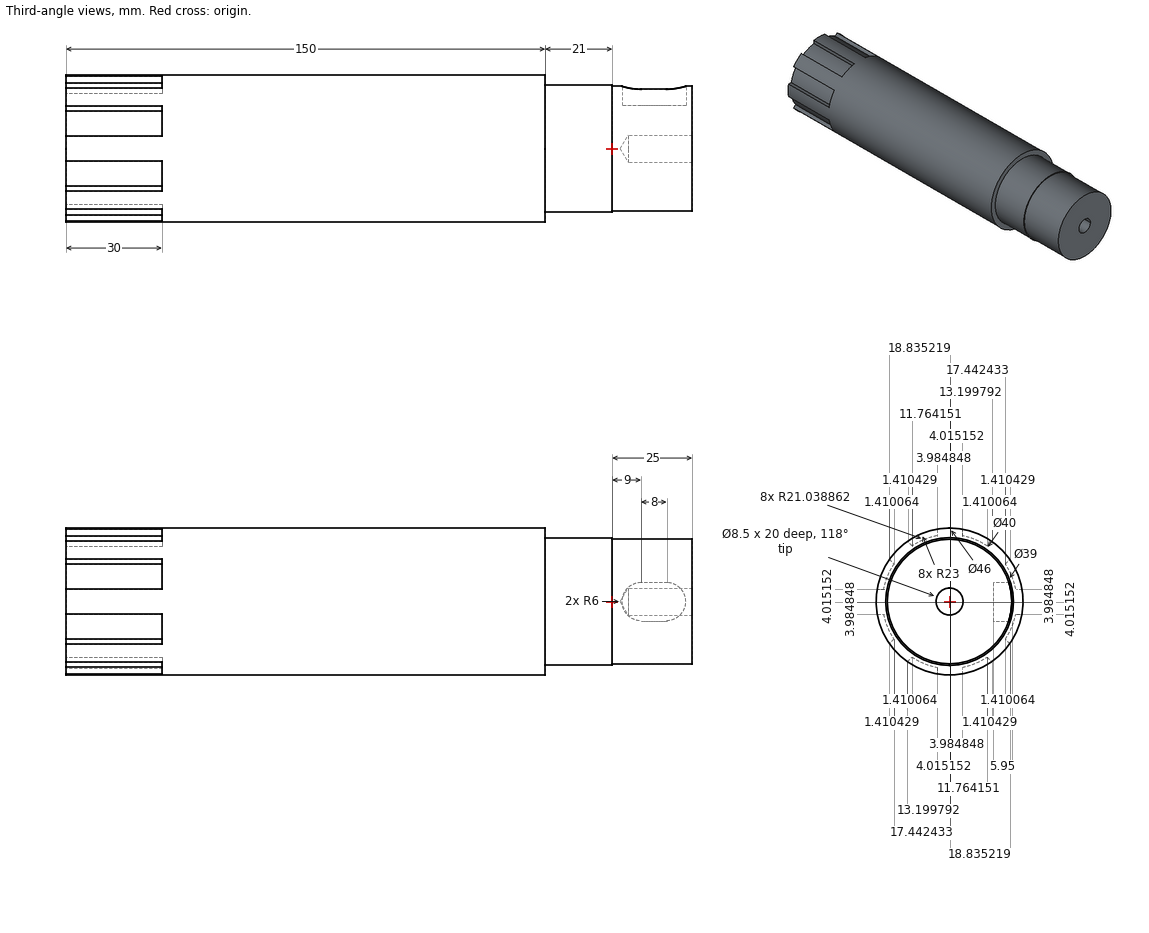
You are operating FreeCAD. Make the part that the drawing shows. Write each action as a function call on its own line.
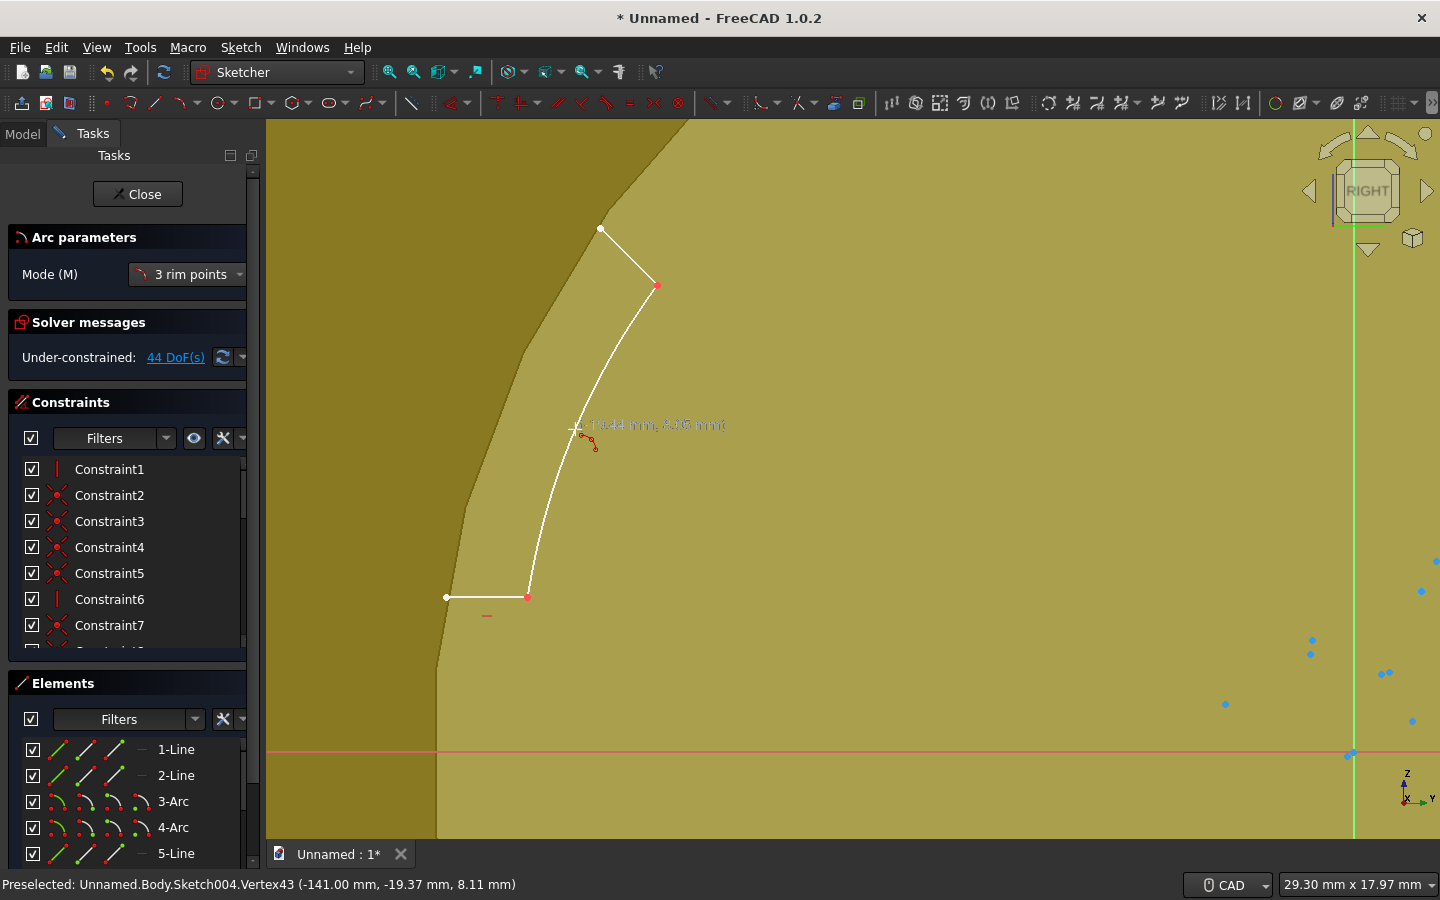
click(447, 597)
click(601, 228)
click(503, 399)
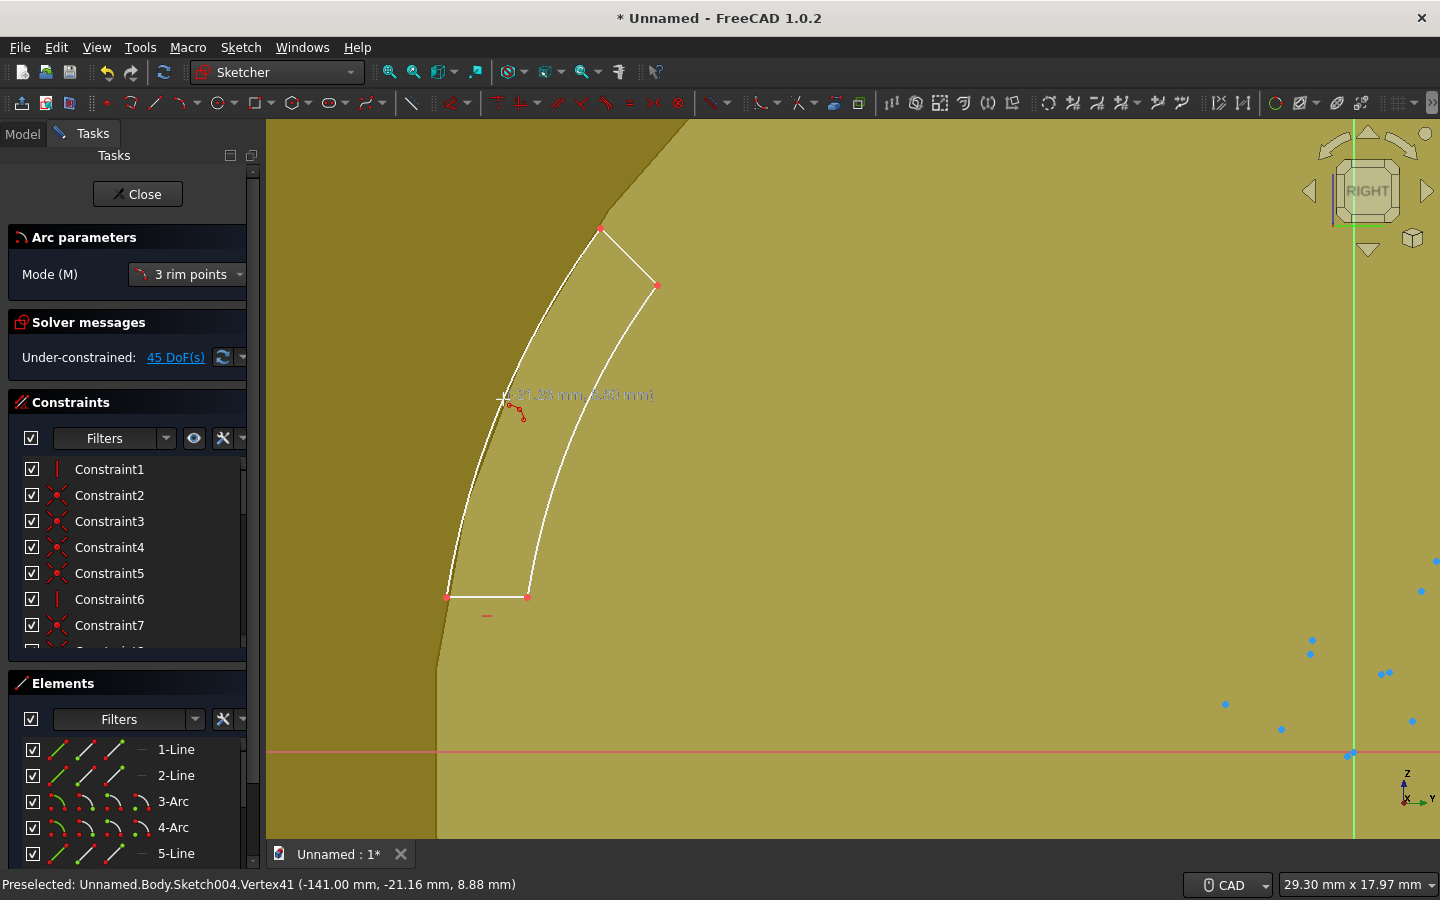
click(156, 104)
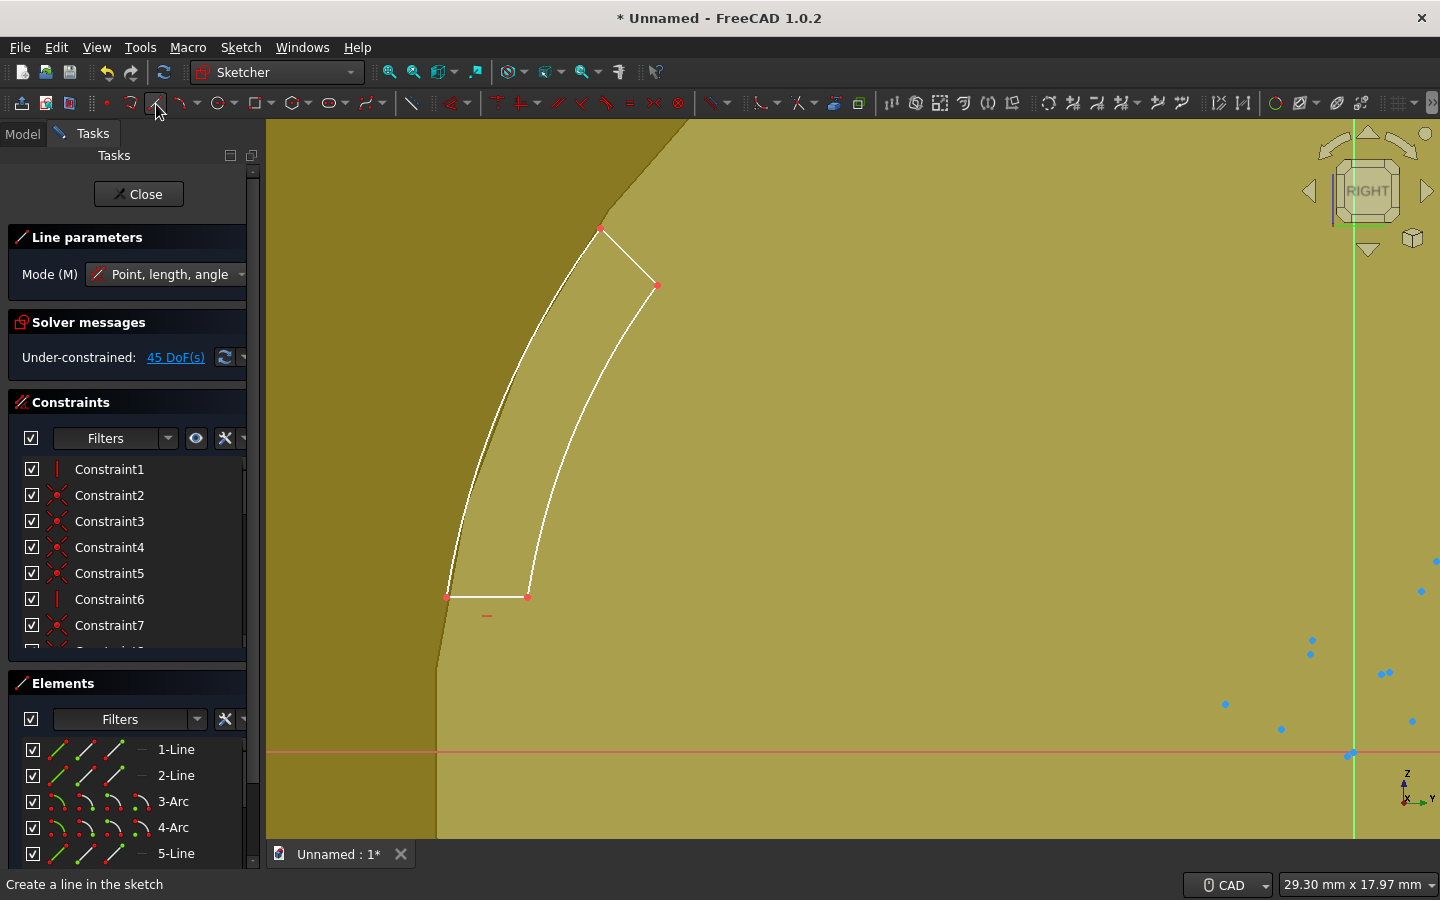
scroll(598, 390, down, 7)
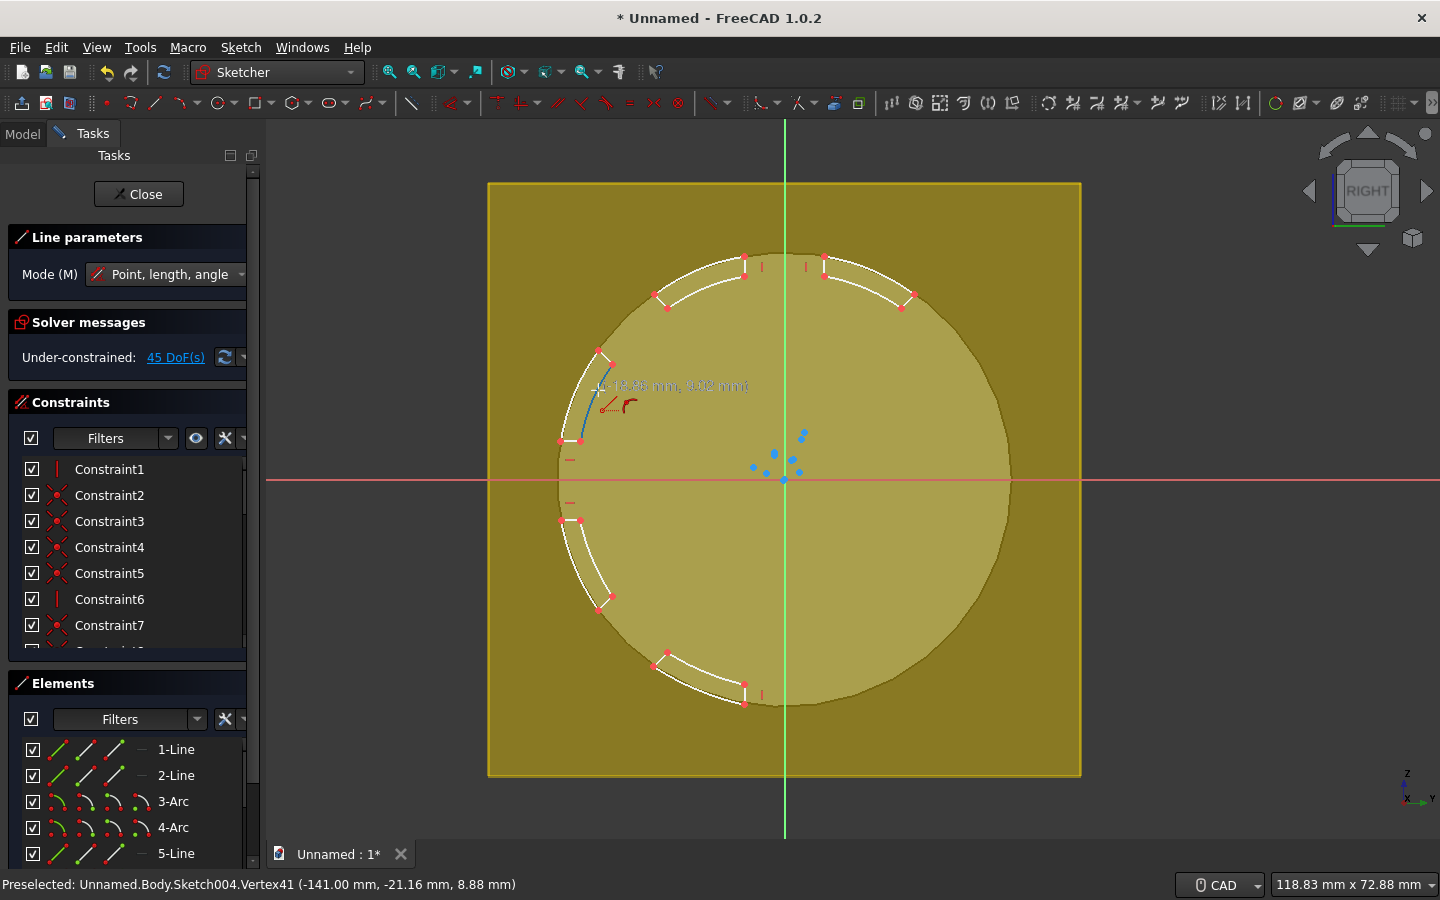
click(1008, 440)
click(989, 440)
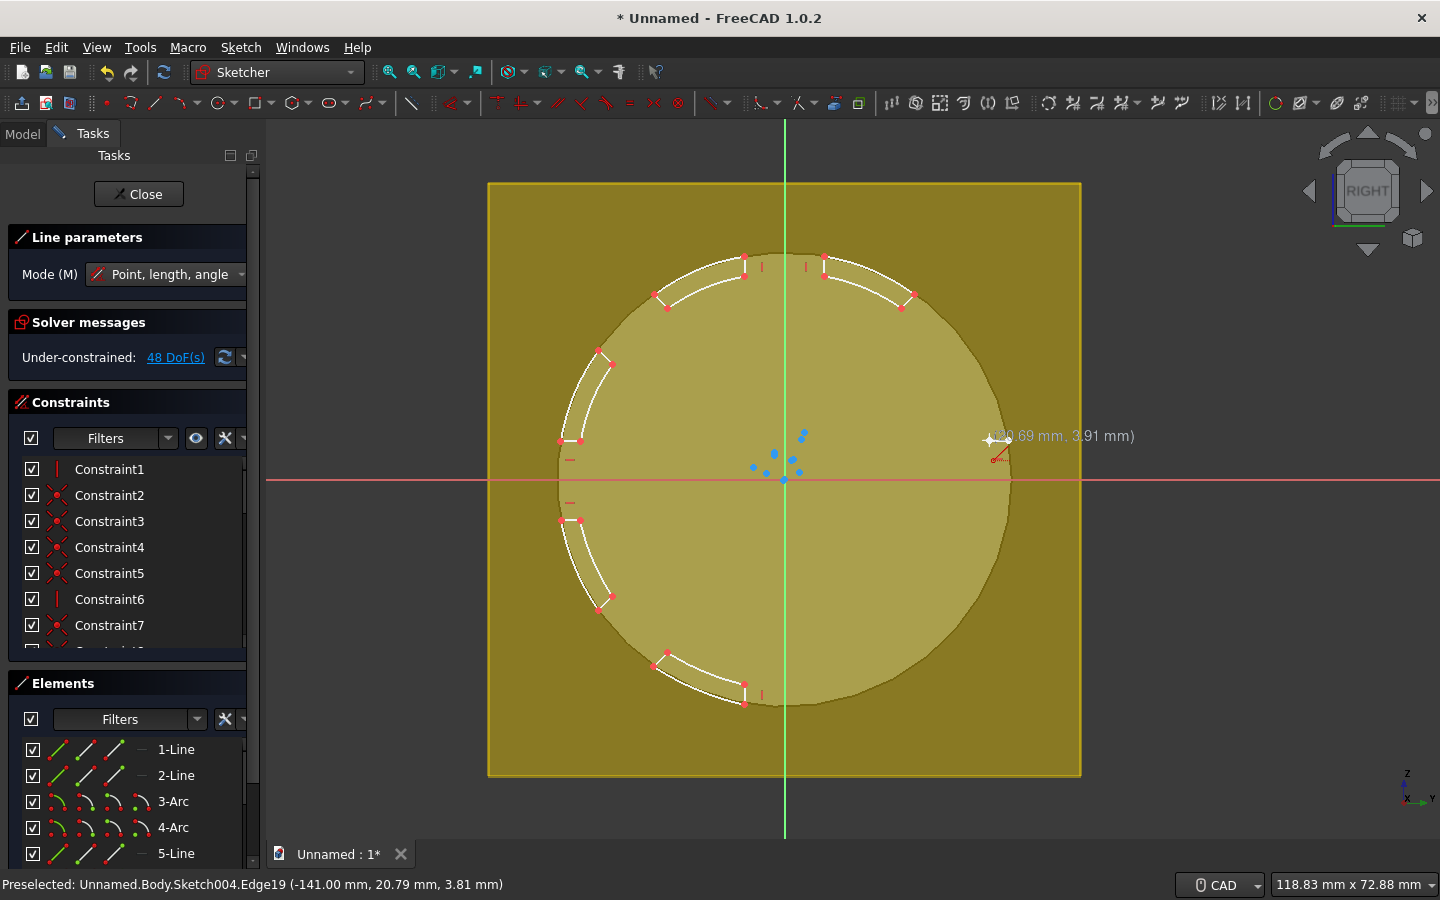
click(957, 363)
click(971, 349)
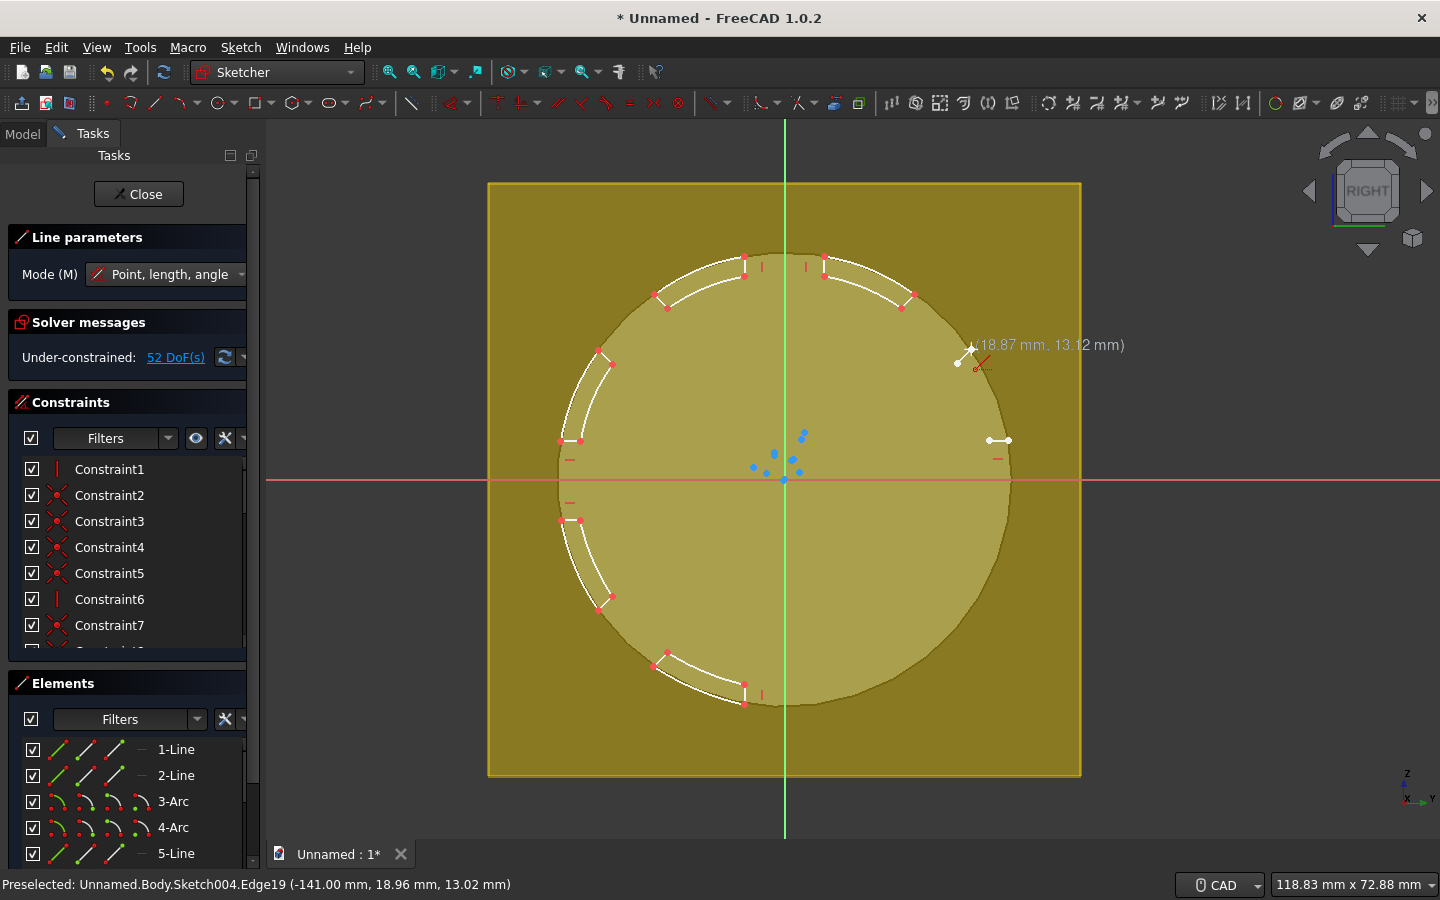
click(180, 104)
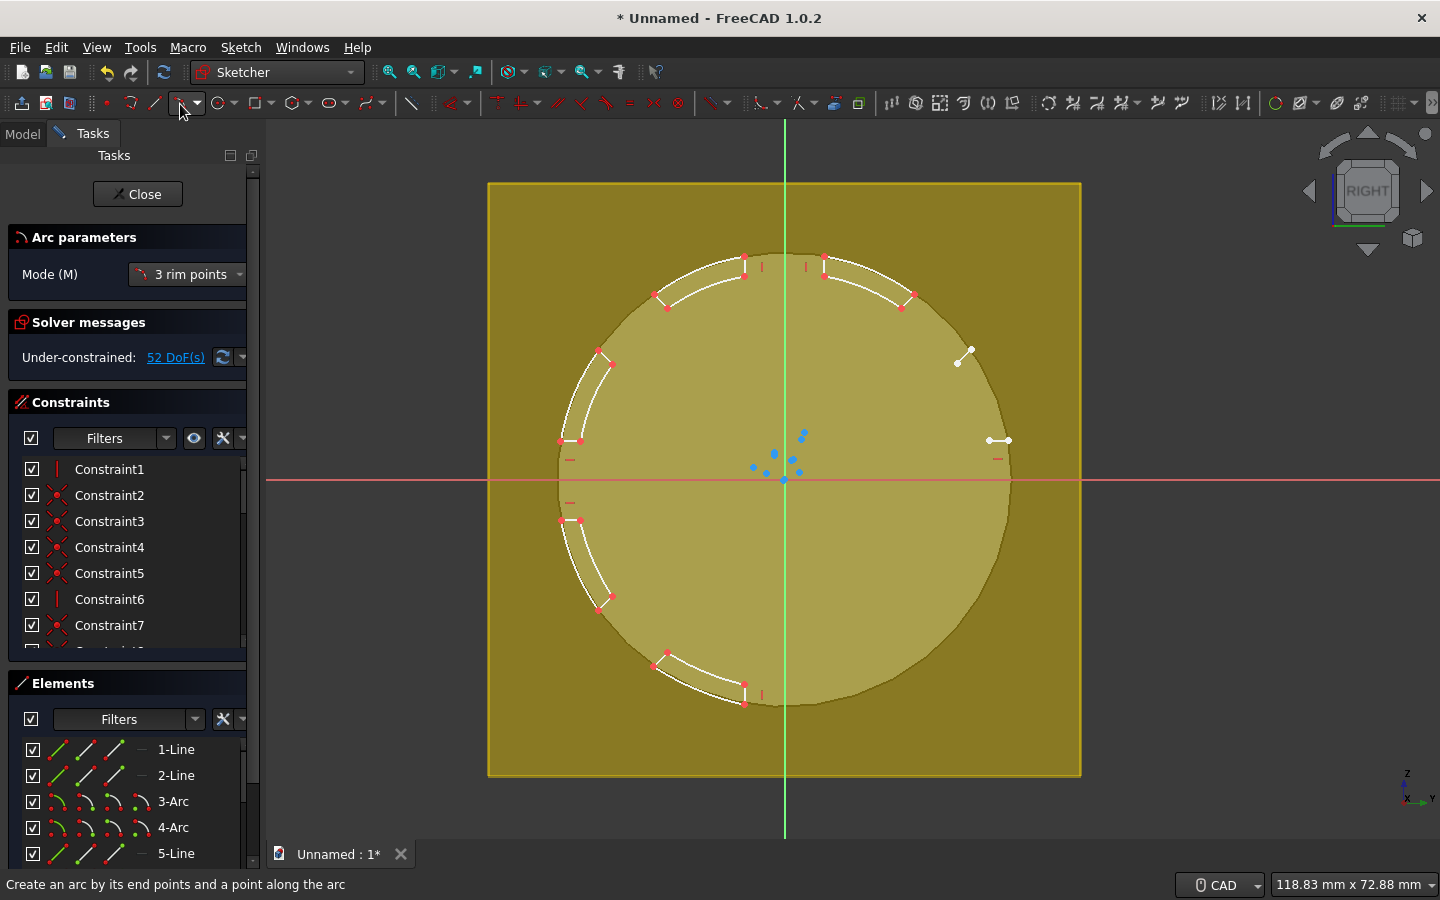
scroll(989, 440, up, 3)